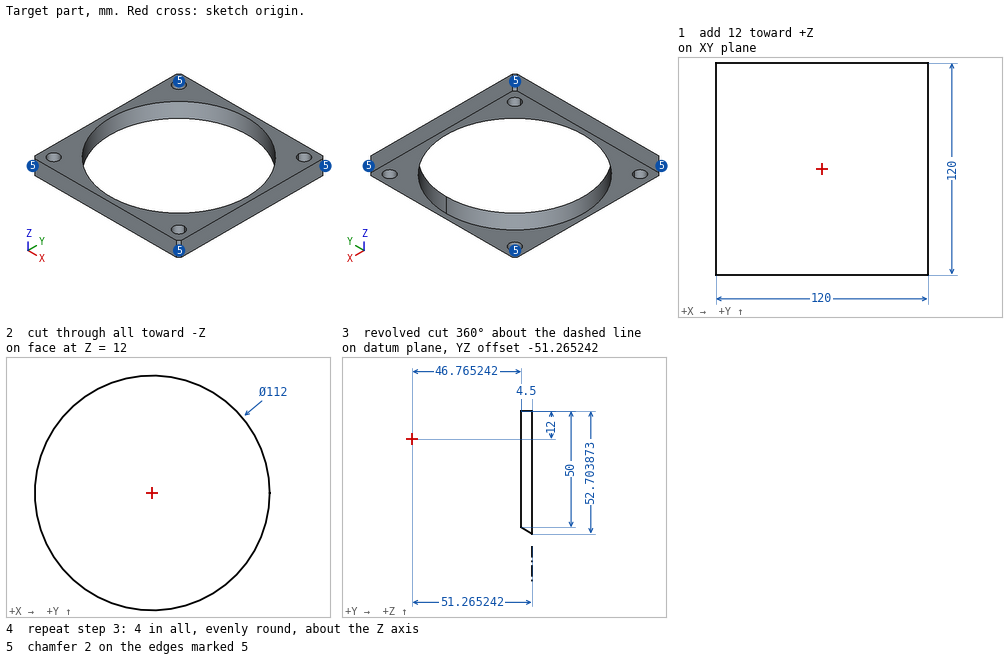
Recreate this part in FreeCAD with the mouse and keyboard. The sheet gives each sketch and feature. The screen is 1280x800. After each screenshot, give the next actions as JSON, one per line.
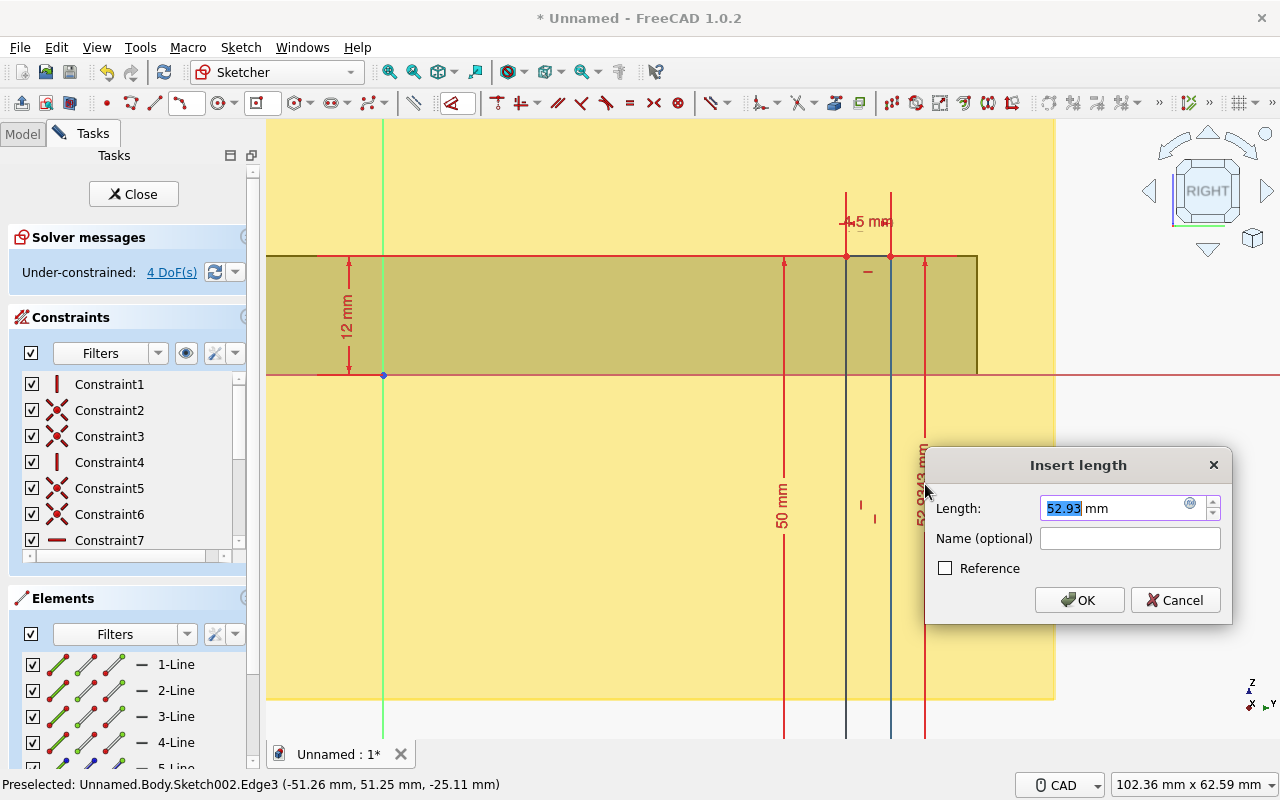
{"action": "type", "text": "52.703873"}
{"action": "key", "text": "Return"}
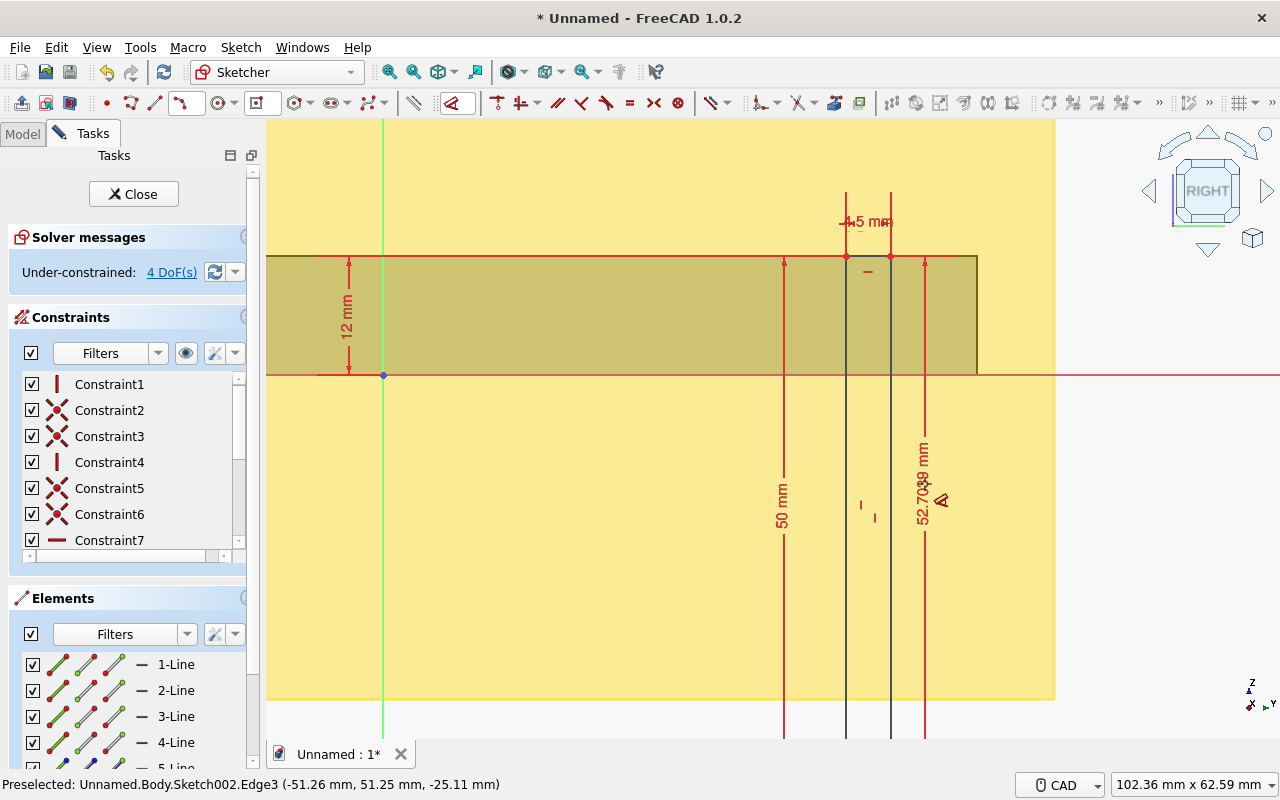
{"action": "left_click", "coordinate": [846, 256]}
{"action": "left_click", "coordinate": [615, 222]}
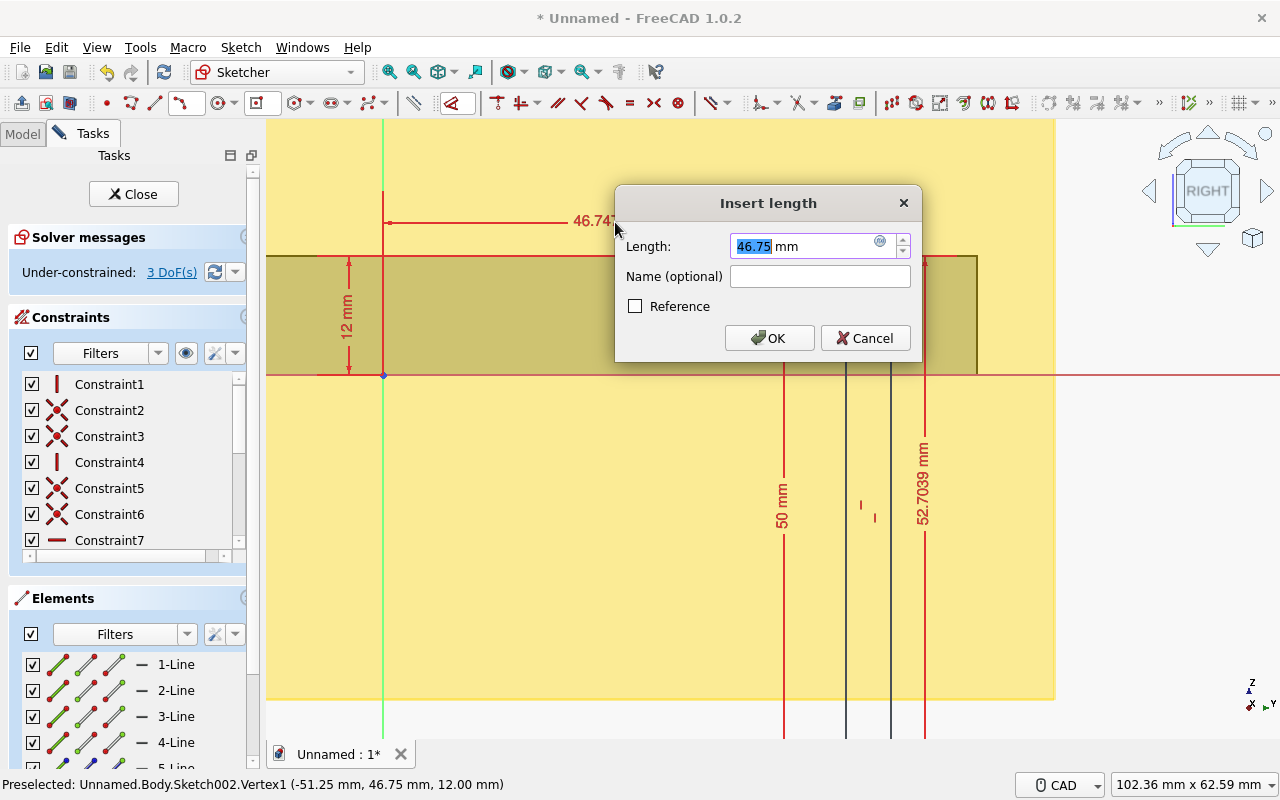
{"action": "type", "text": "46.765242"}
{"action": "key", "text": "Return"}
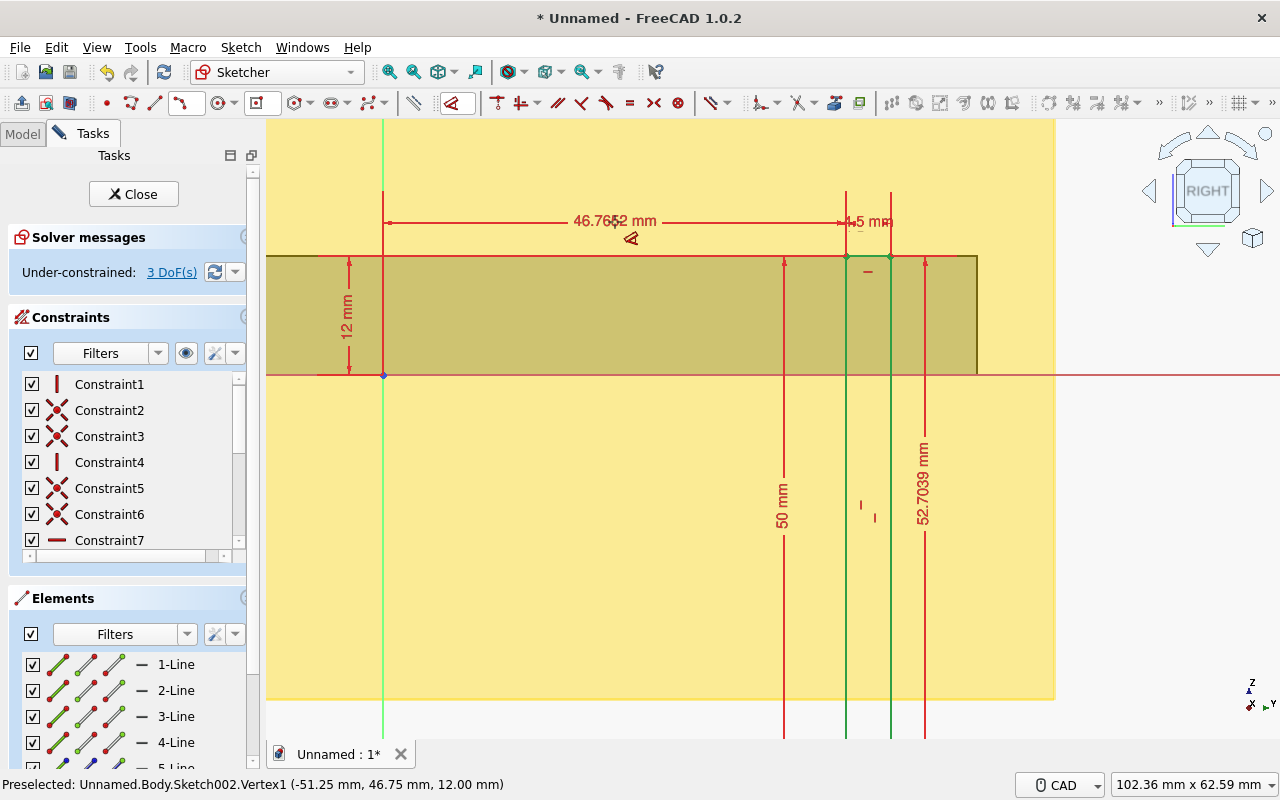
{"action": "scroll", "coordinate": [787, 194], "scroll_direction": "down", "scroll_amount": 3}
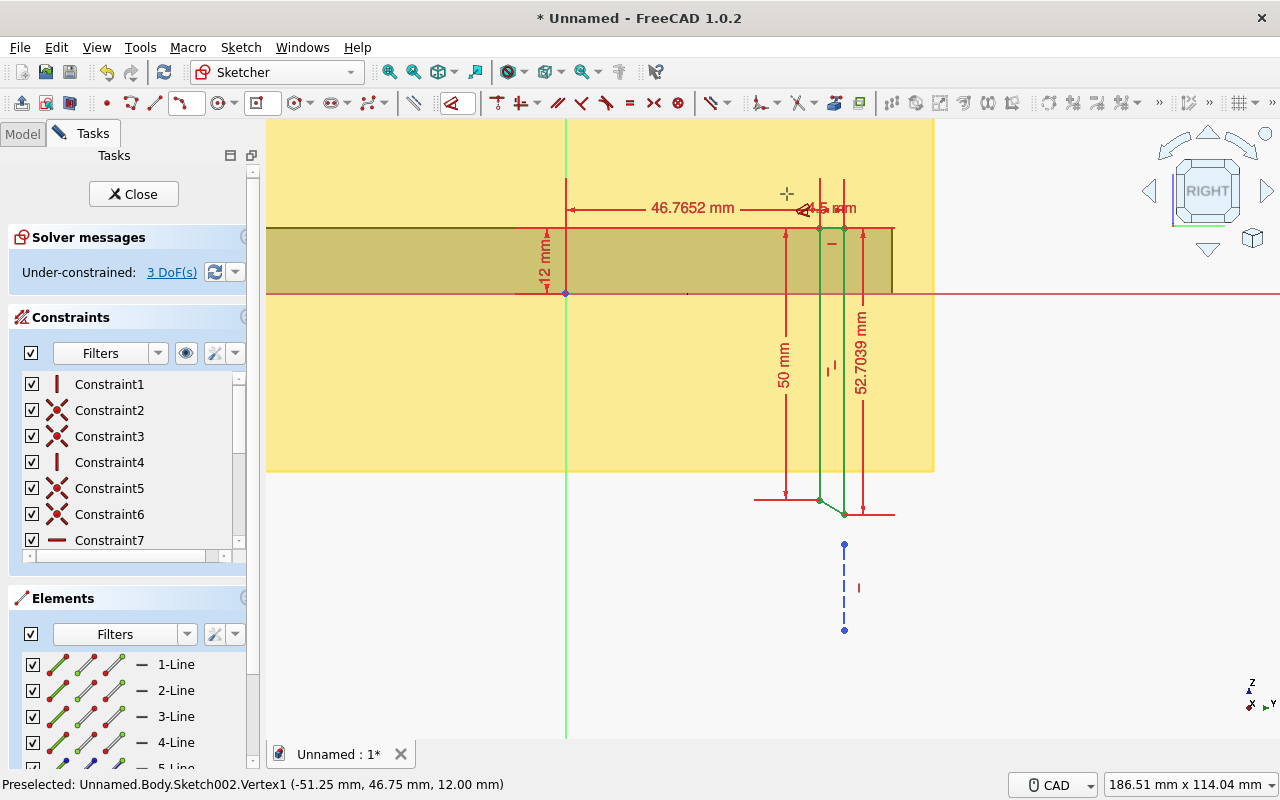
{"action": "left_click", "coordinate": [844, 544]}
{"action": "left_click", "coordinate": [705, 260]}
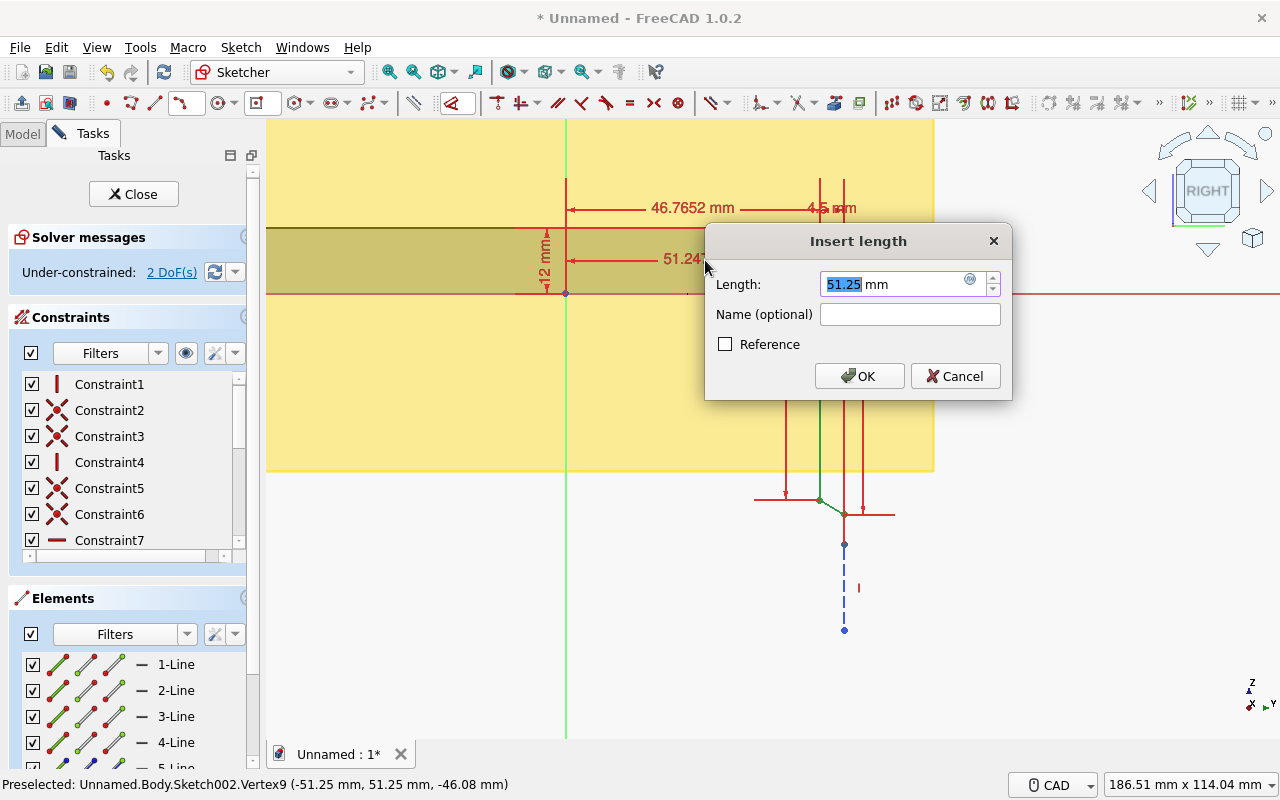
{"action": "type", "text": "51.265242"}
{"action": "key", "text": "Return"}
{"action": "key", "text": "Escape"}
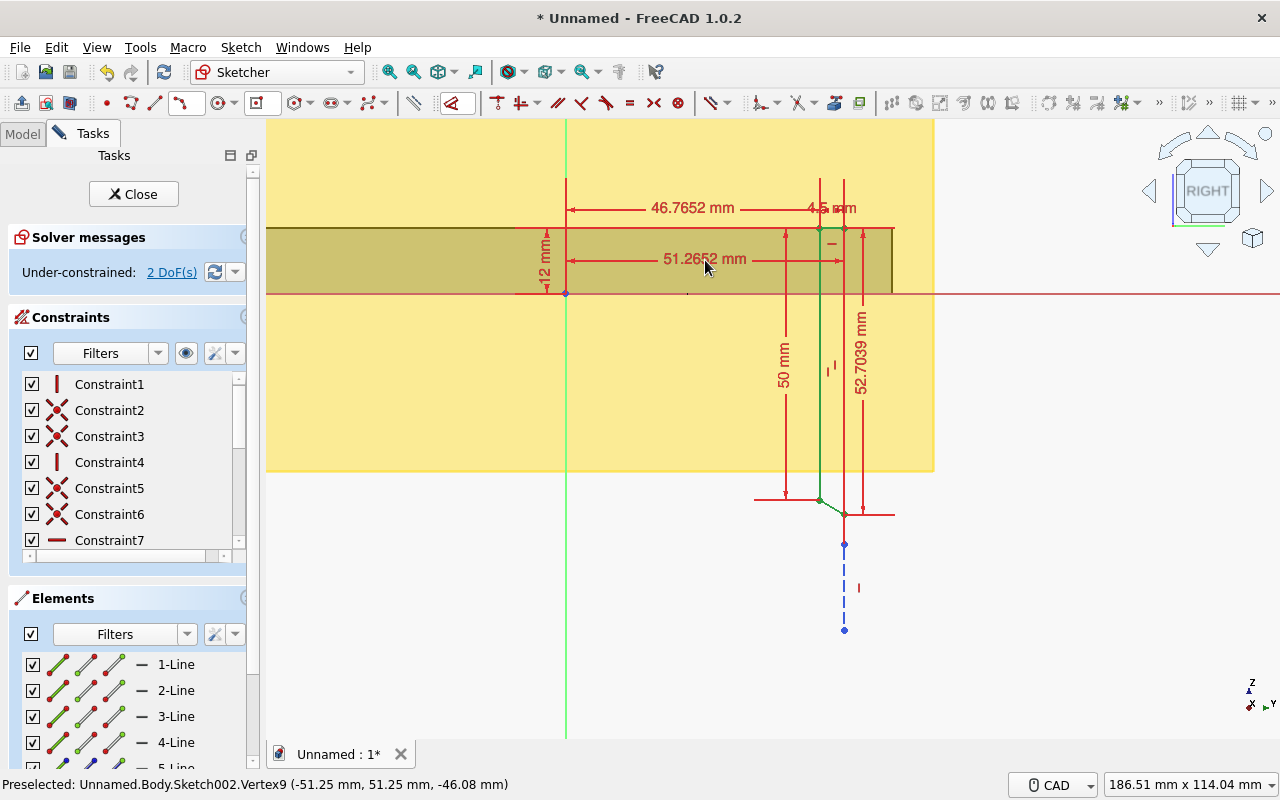
{"action": "left_click", "coordinate": [134, 194]}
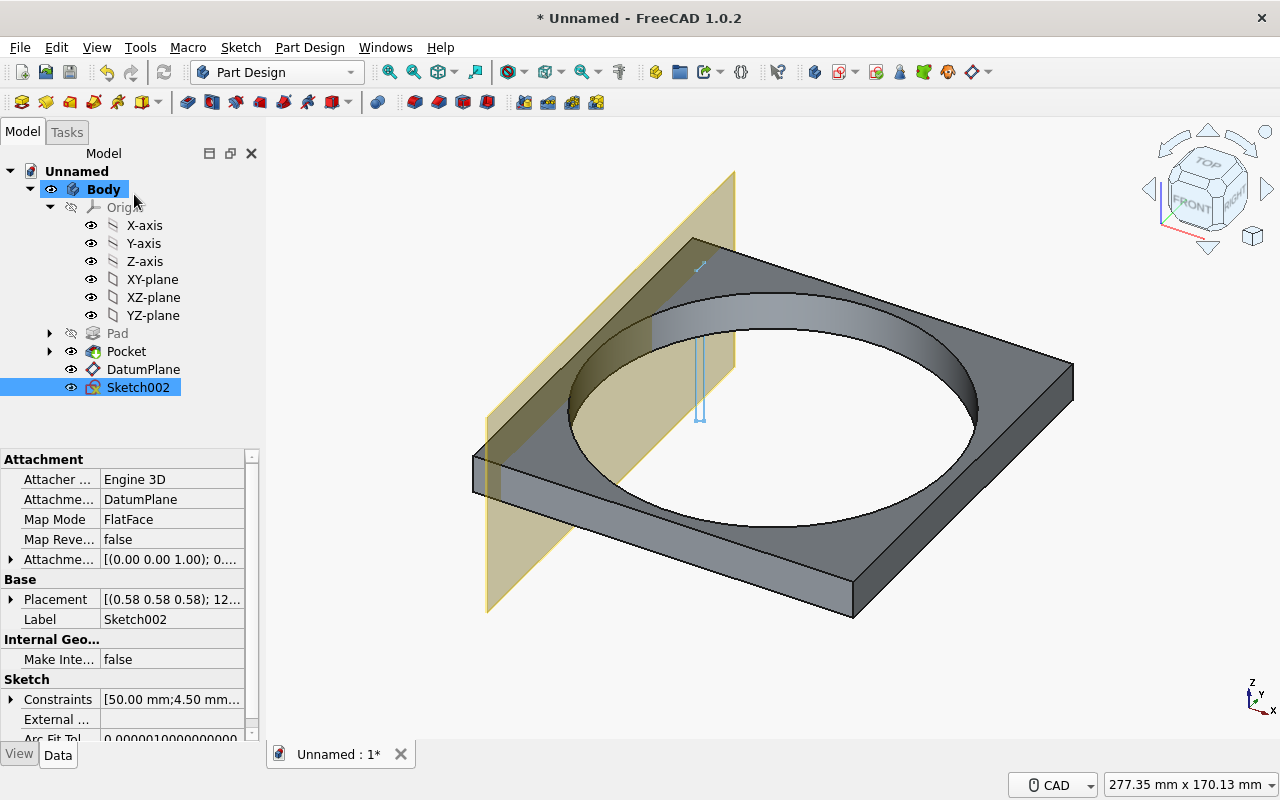
{"action": "left_click", "coordinate": [236, 102]}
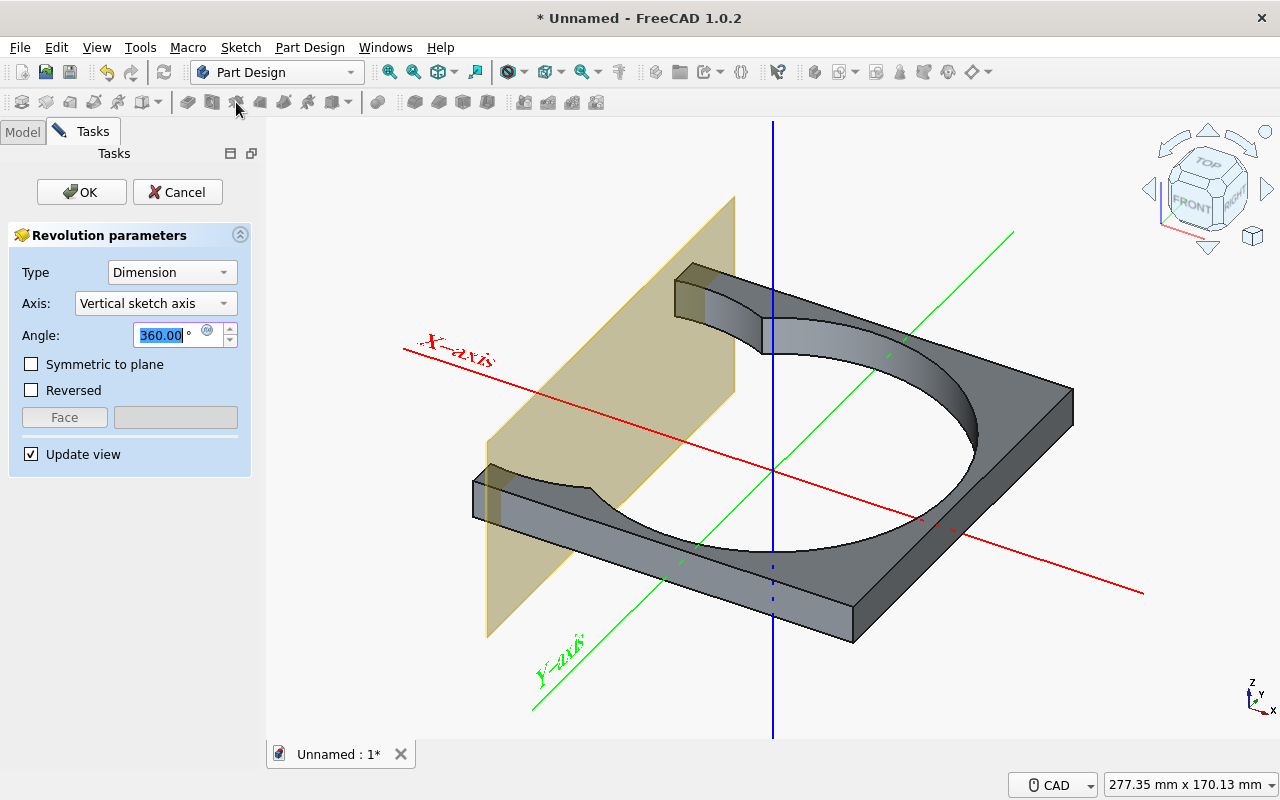
{"action": "left_click", "coordinate": [156, 304]}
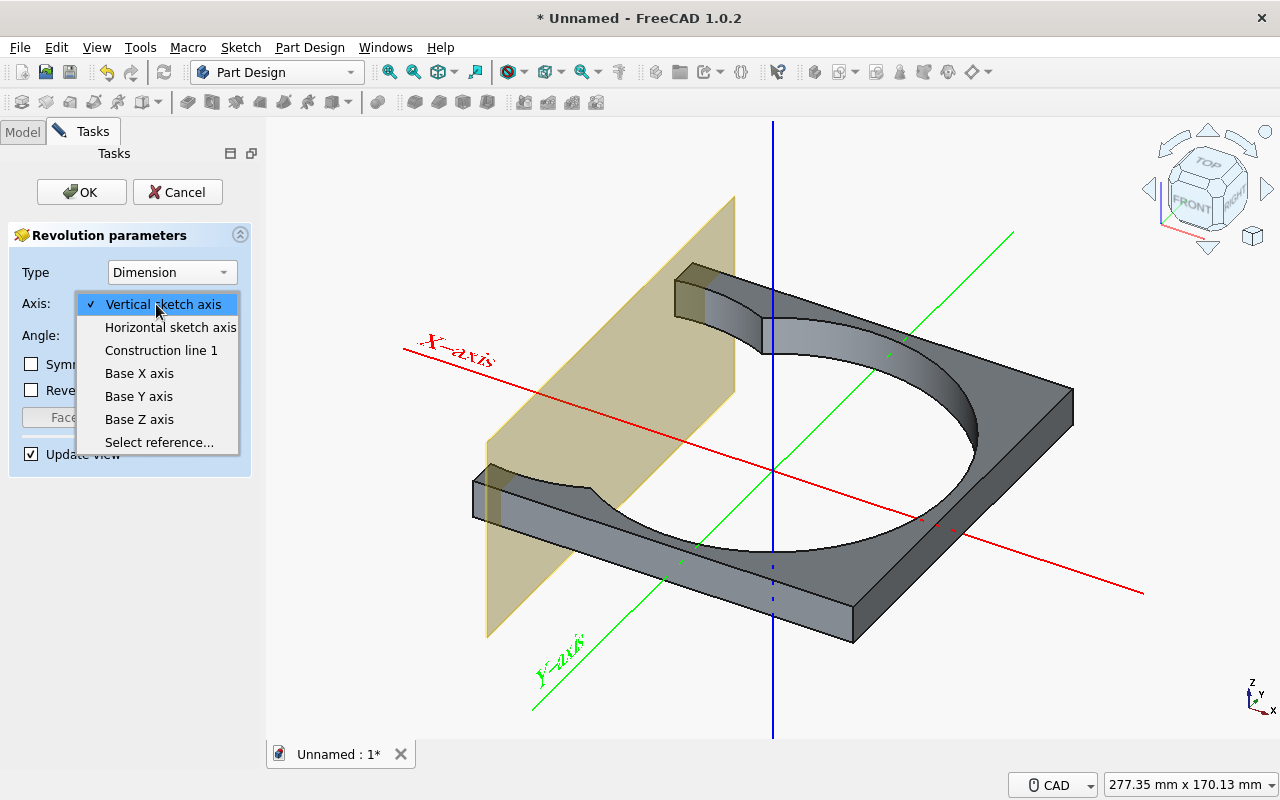
{"action": "left_click", "coordinate": [156, 350]}